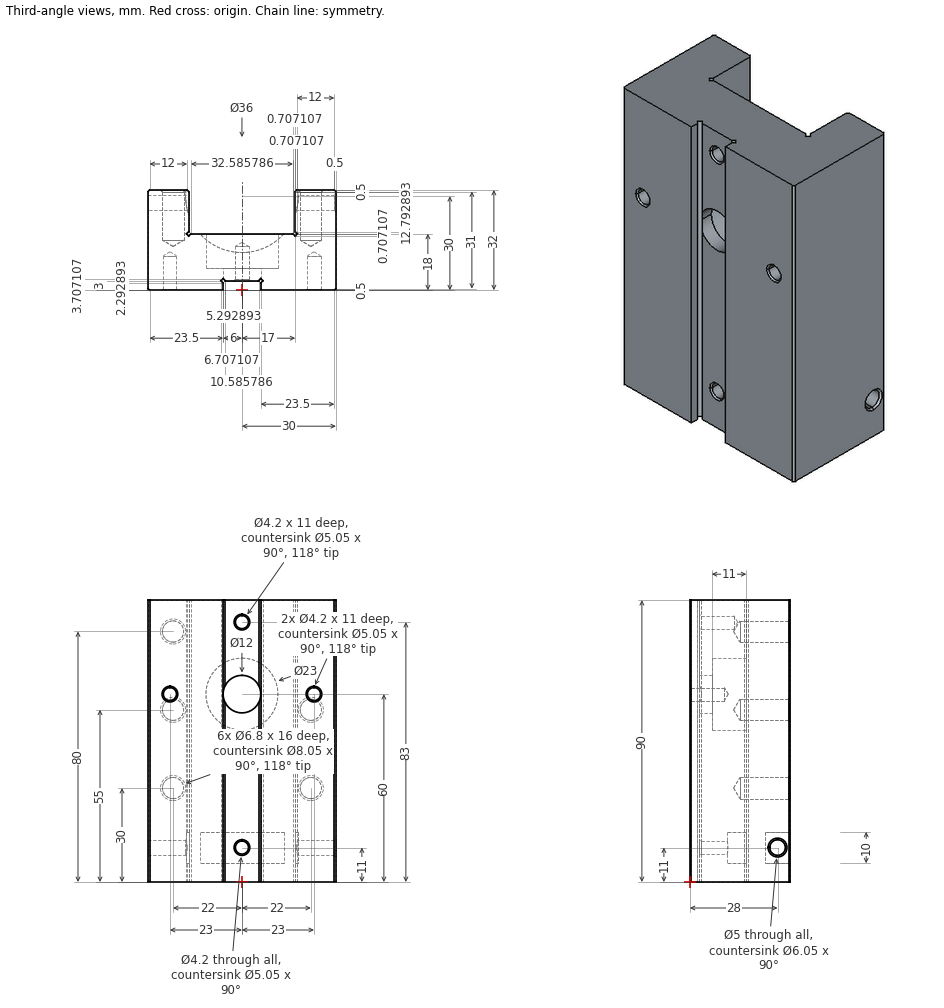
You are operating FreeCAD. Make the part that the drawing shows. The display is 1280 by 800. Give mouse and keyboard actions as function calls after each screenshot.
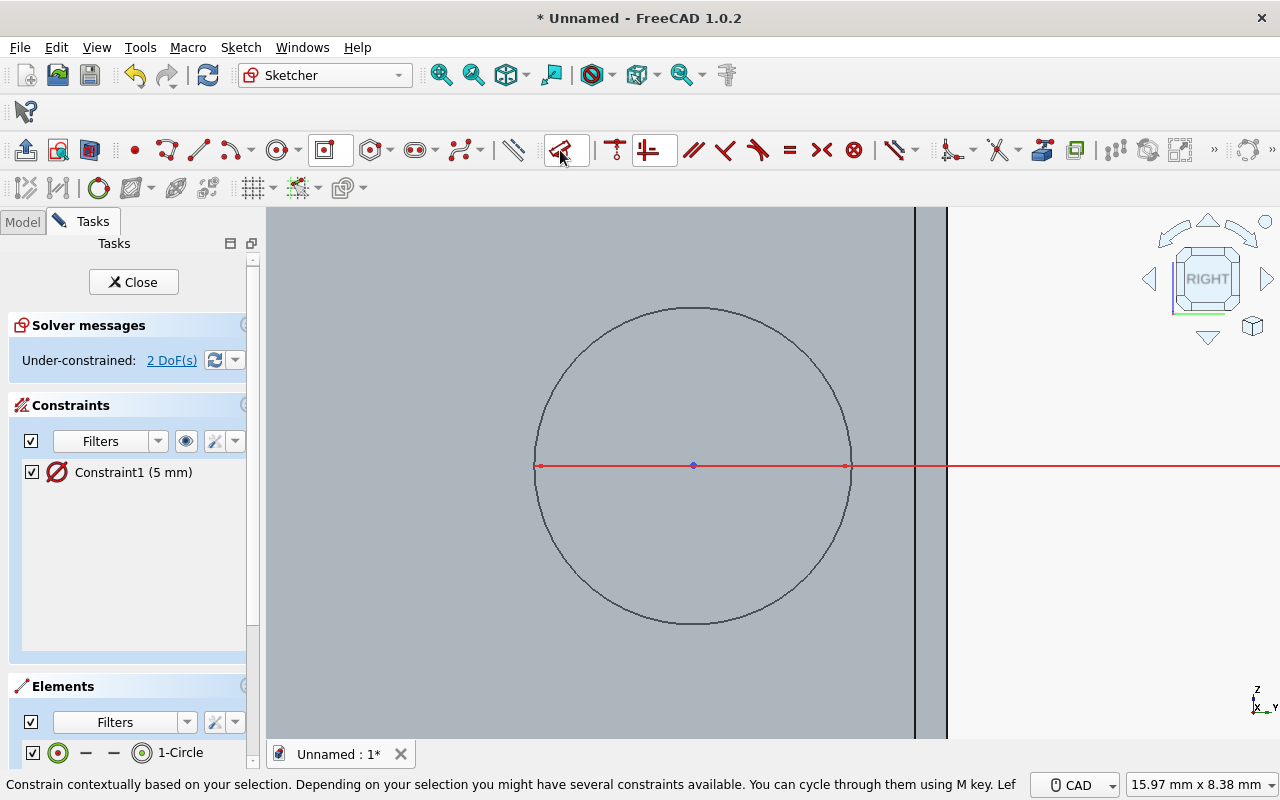
click(693, 466)
click(494, 432)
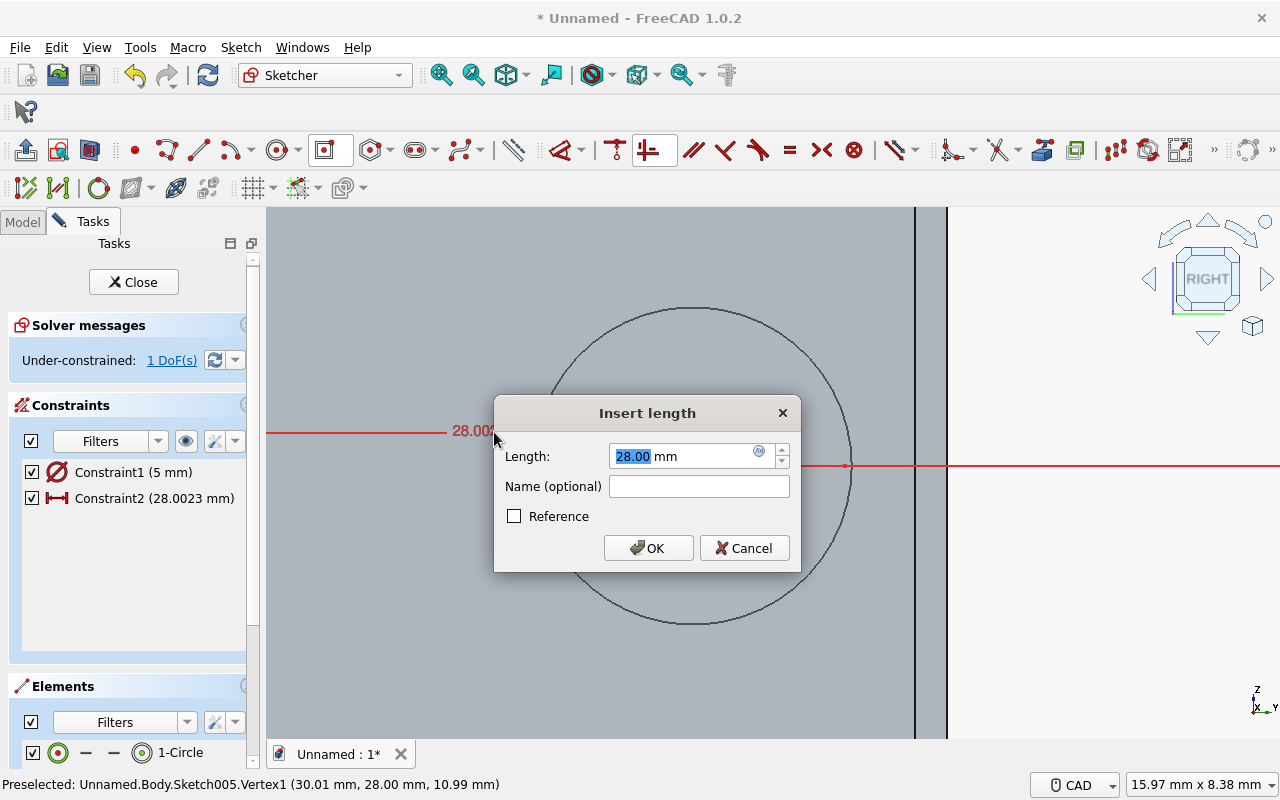
text(28)
key(Return)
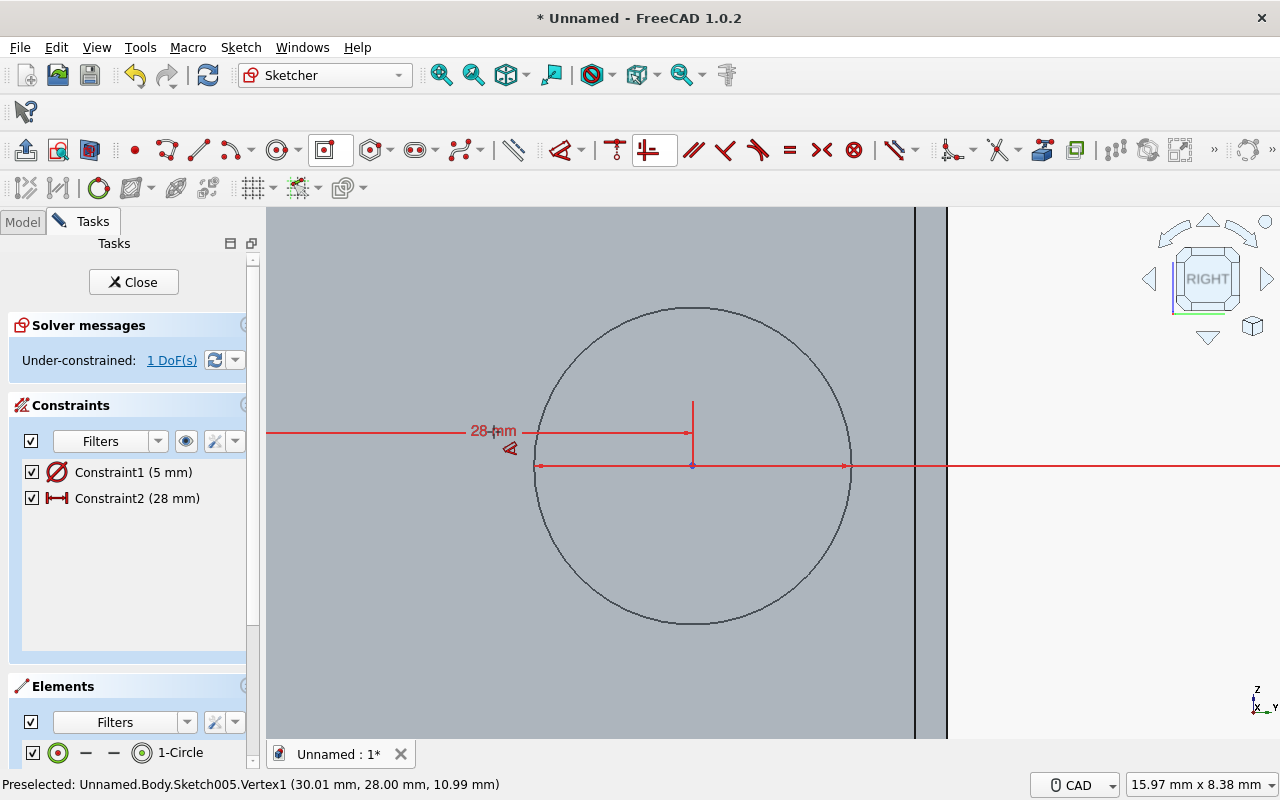
click(693, 466)
click(727, 589)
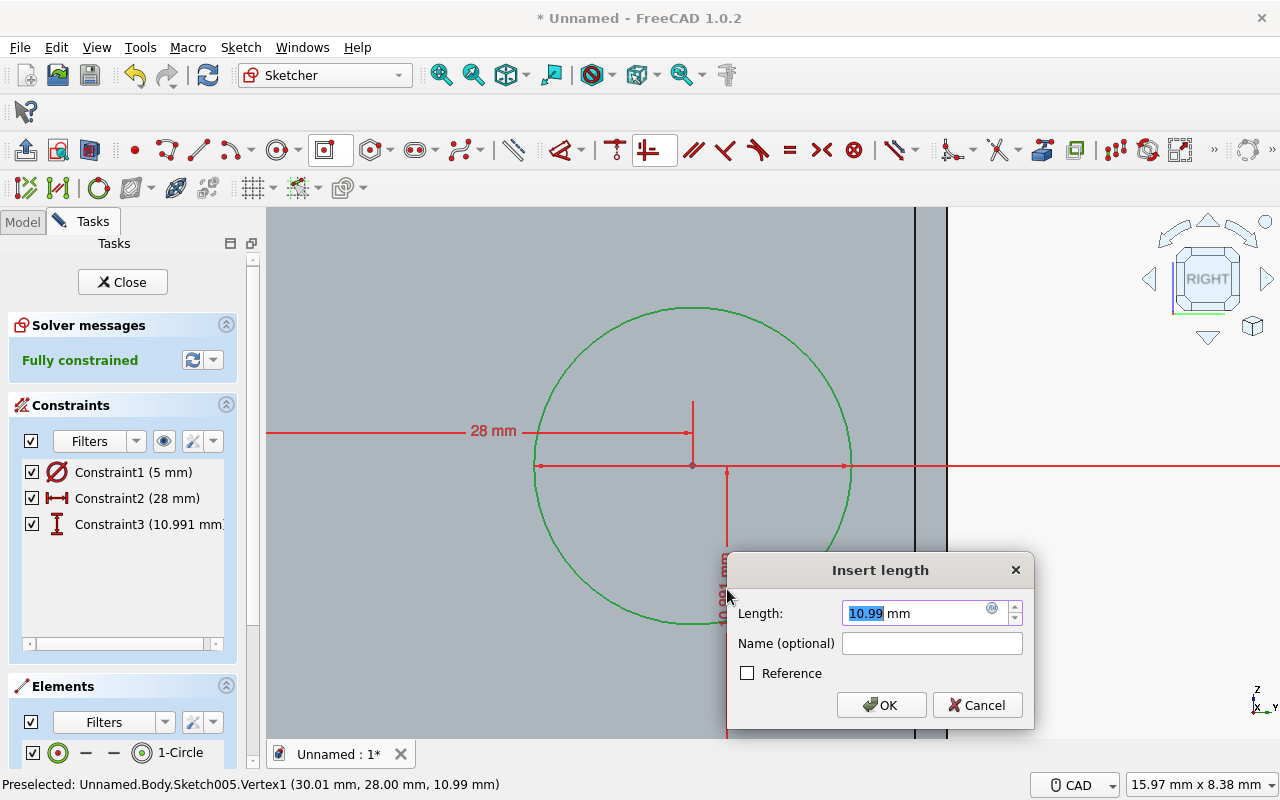
text(11)
key(Return)
key(Escape)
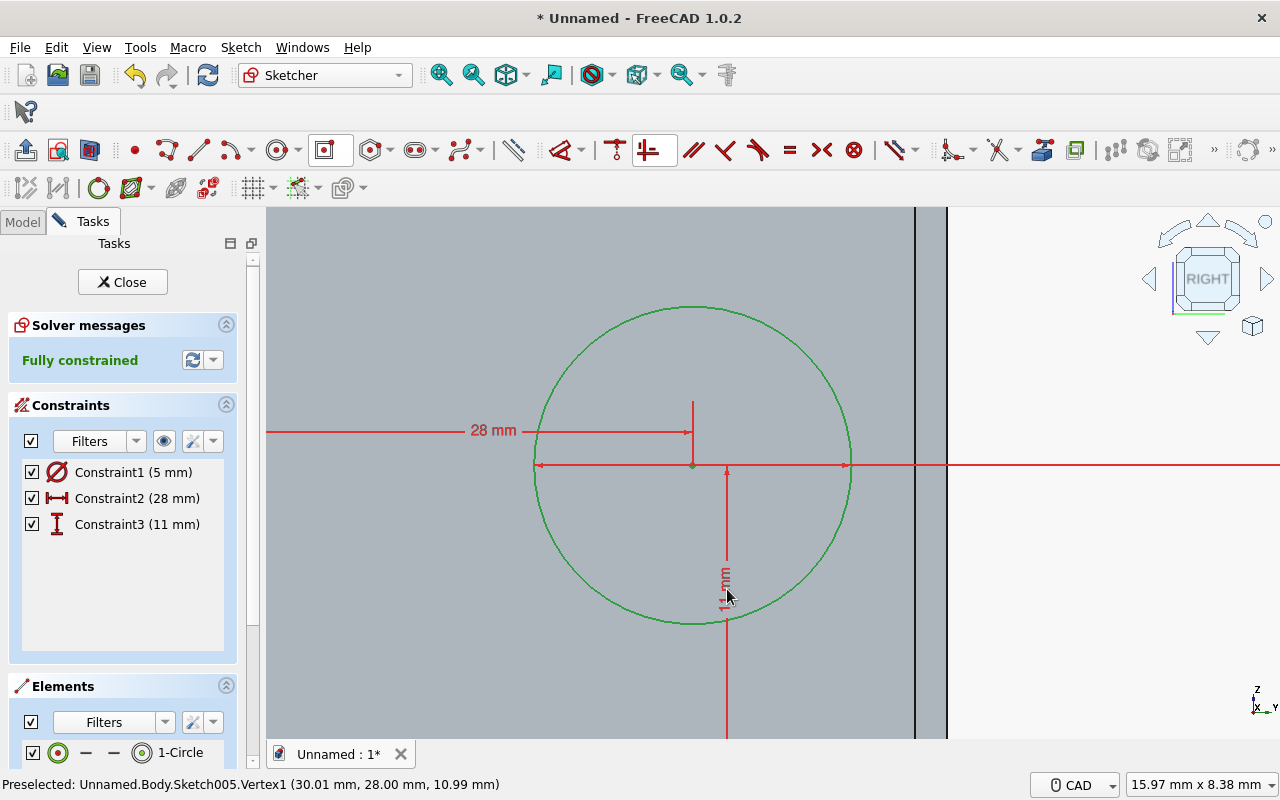
click(123, 282)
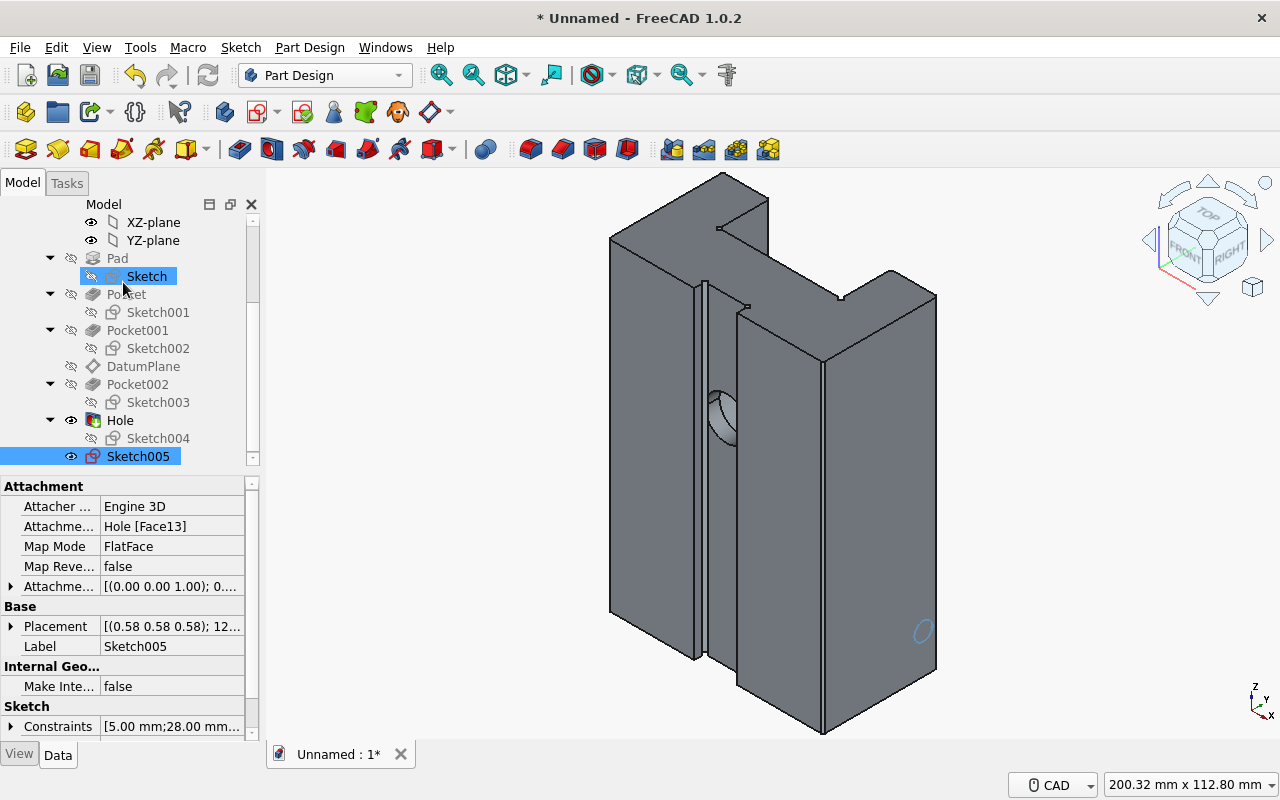
click(272, 150)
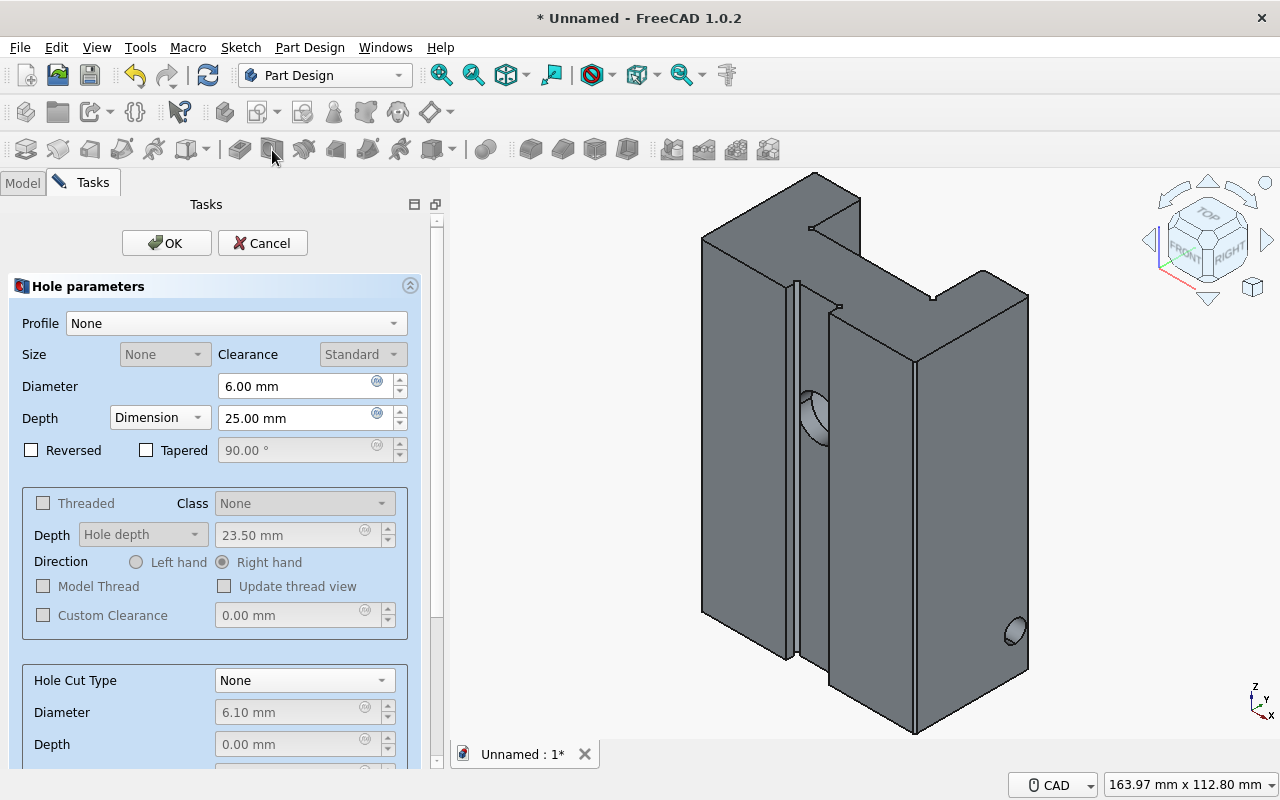
triple_click(305, 386)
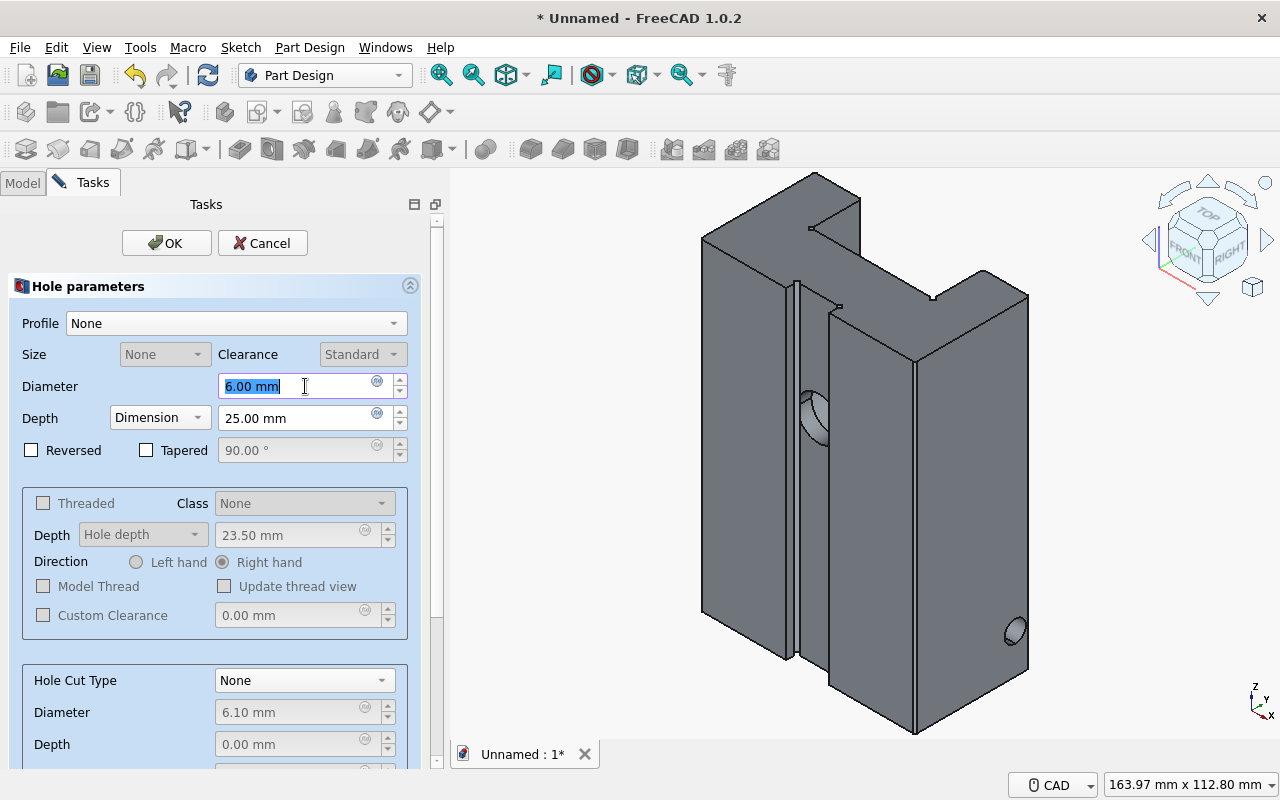
text(5)
key(Tab)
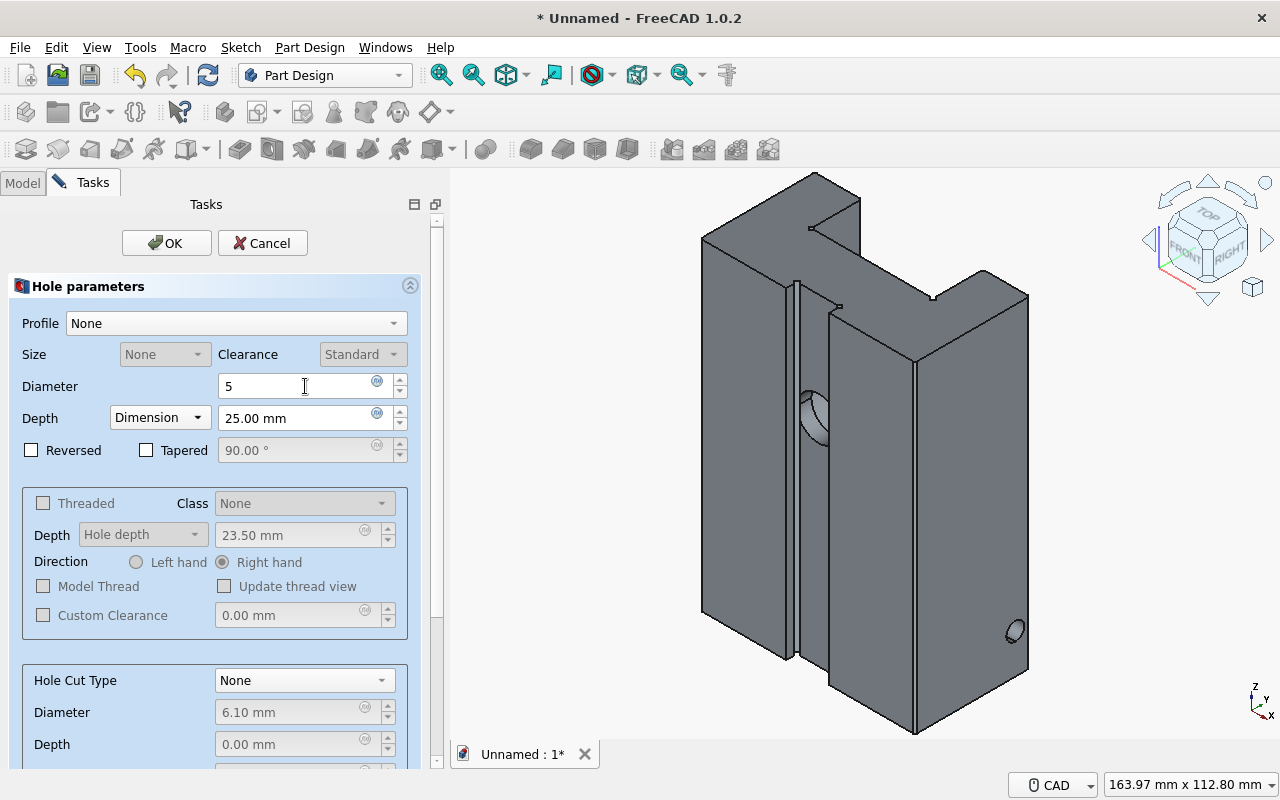
click(161, 418)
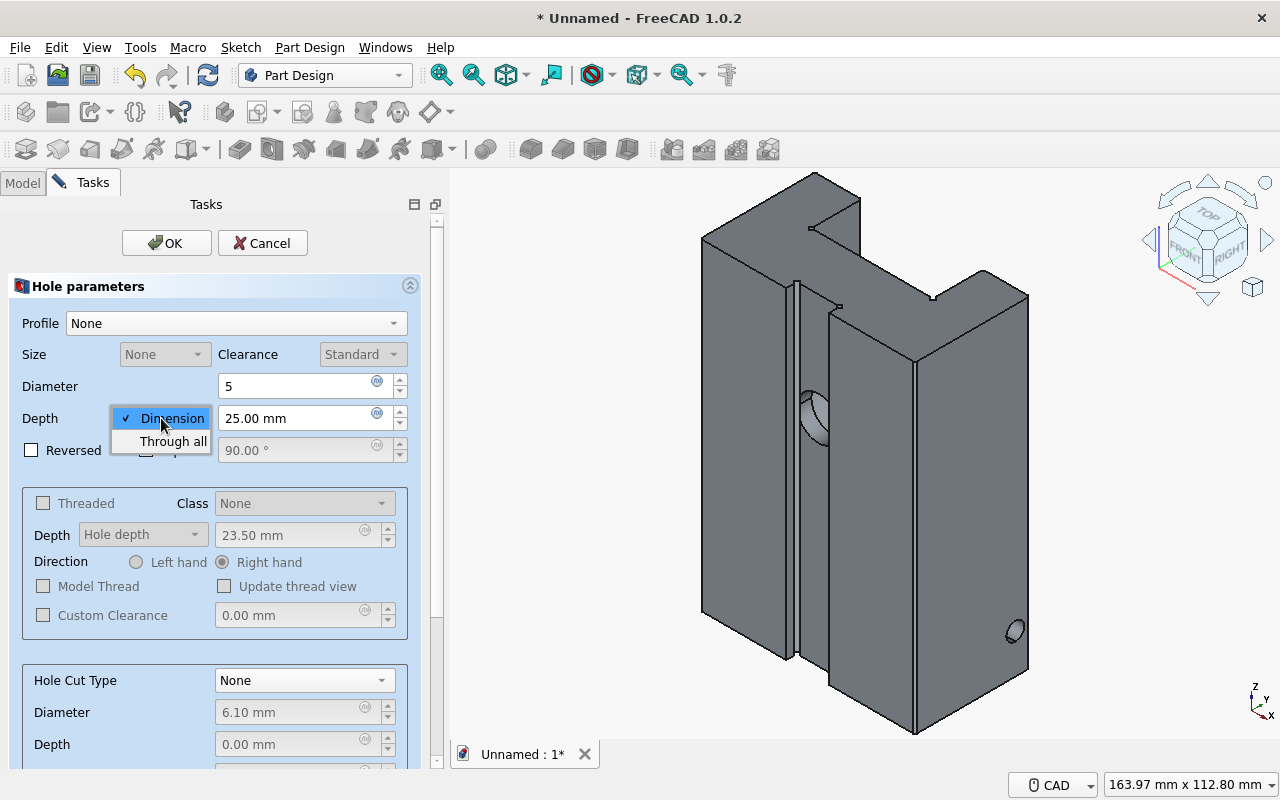
click(160, 442)